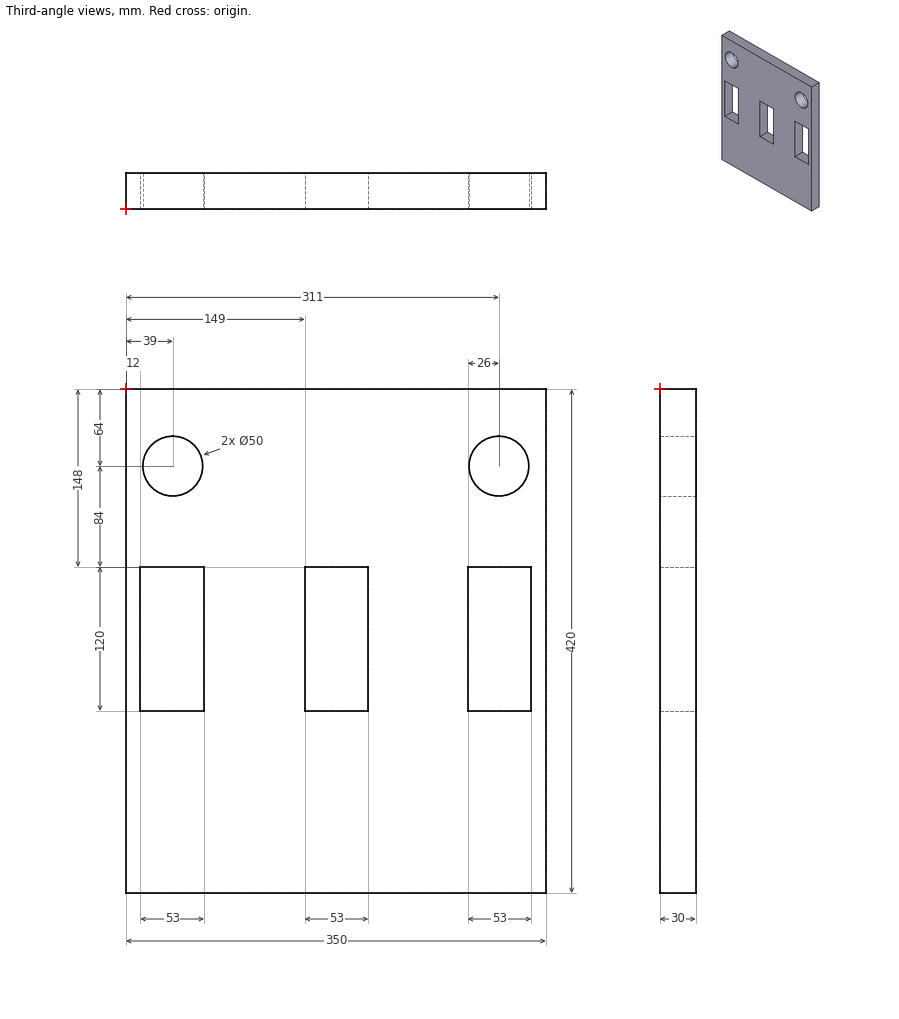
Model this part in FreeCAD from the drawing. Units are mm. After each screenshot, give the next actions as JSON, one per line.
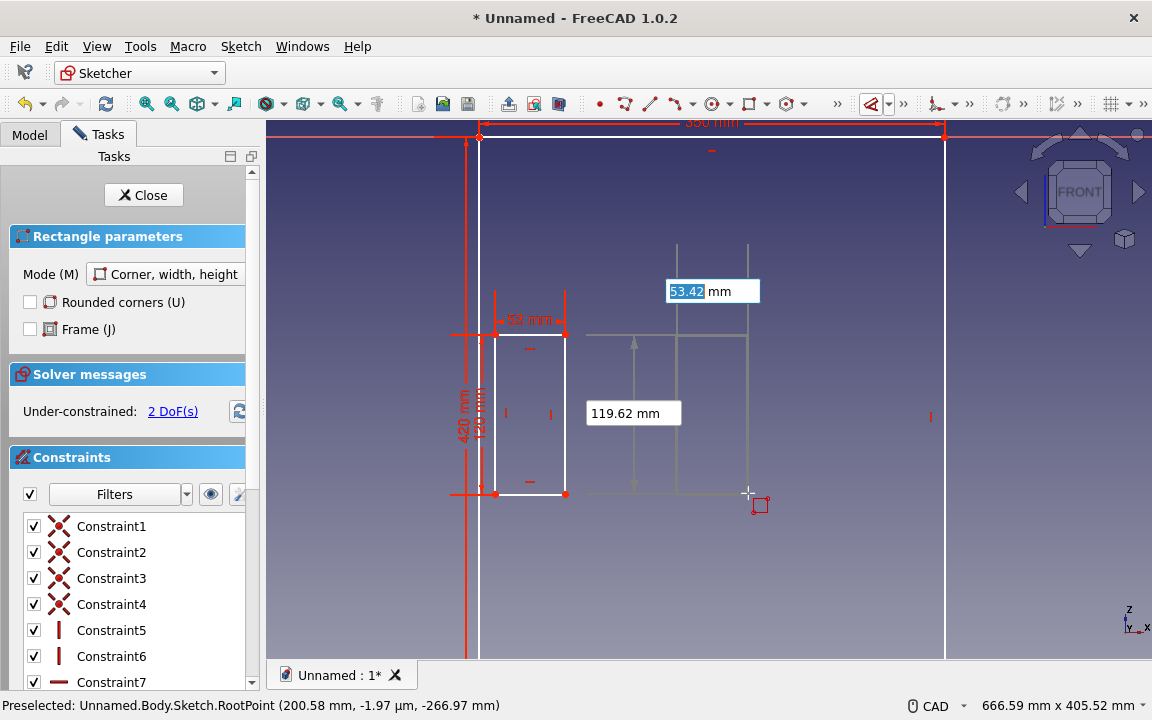
{"action": "type", "text": "53"}
{"action": "key", "text": "Tab"}
{"action": "type", "text": "120"}
{"action": "key", "text": "Return"}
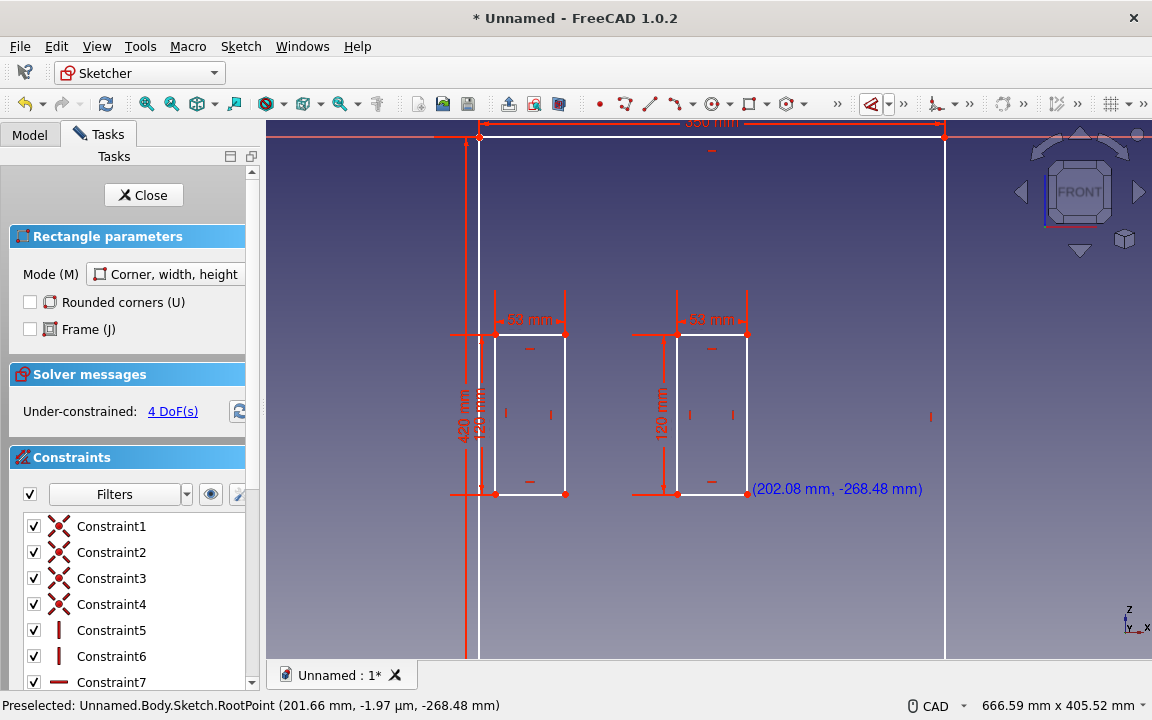
{"action": "left_click", "coordinate": [858, 334]}
{"action": "mouse_move", "coordinate": [929, 493]}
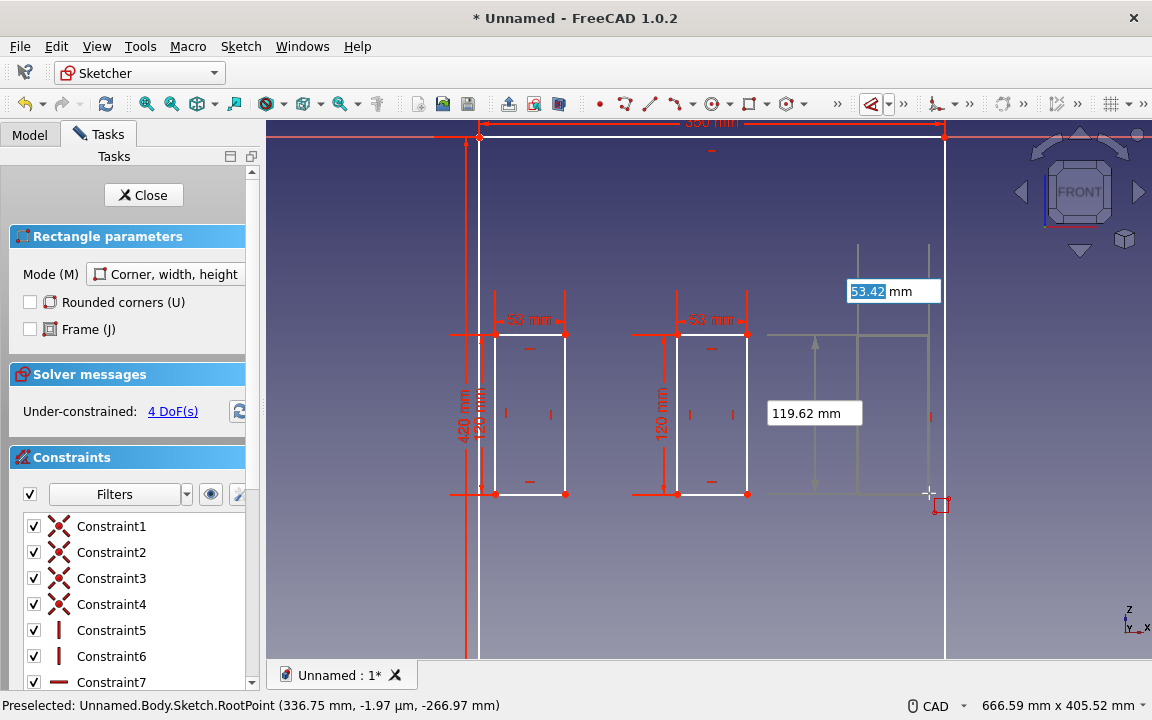
{"action": "type", "text": "53"}
{"action": "key", "text": "Tab"}
{"action": "type", "text": "120"}
{"action": "key", "text": "Return"}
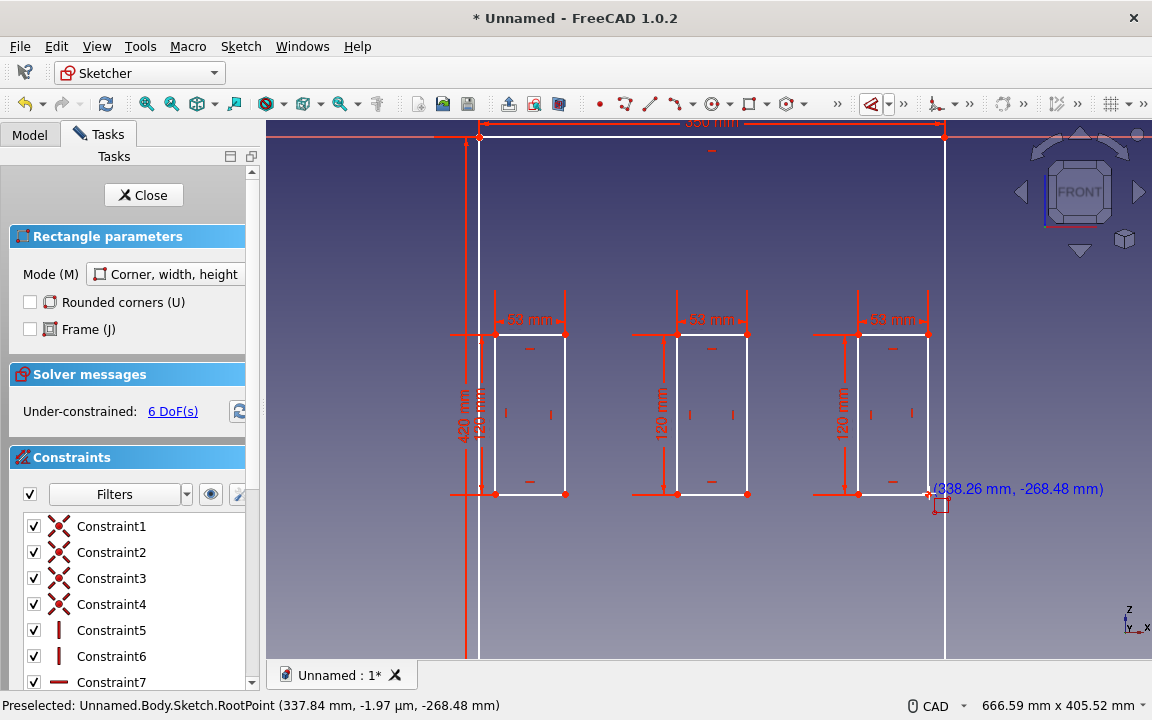
{"action": "left_click", "coordinate": [712, 104]}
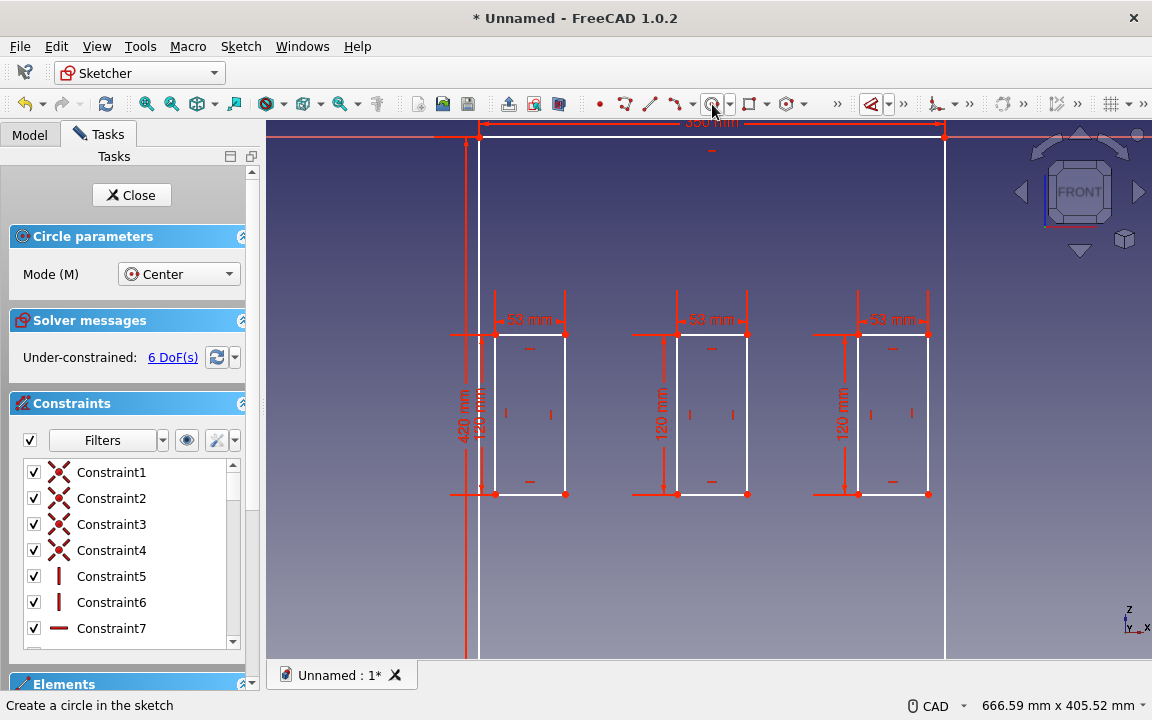
{"action": "left_click", "coordinate": [531, 222]}
{"action": "mouse_move", "coordinate": [555, 199]}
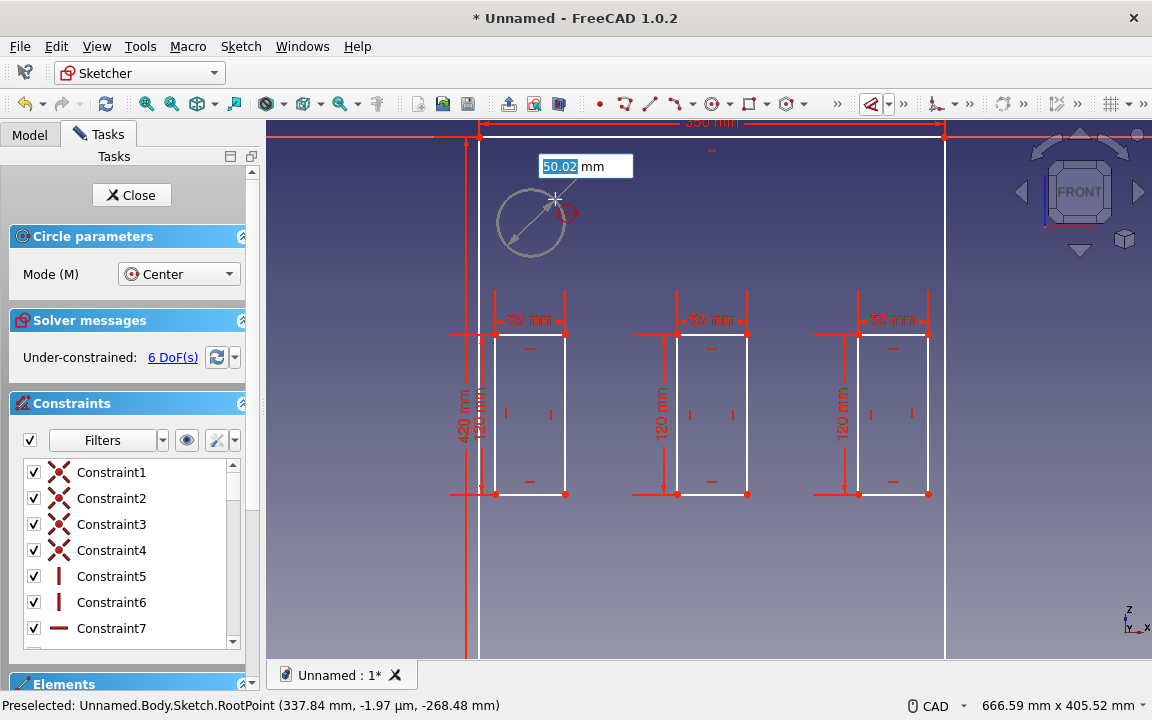
{"action": "type", "text": "50"}
{"action": "key", "text": "Return"}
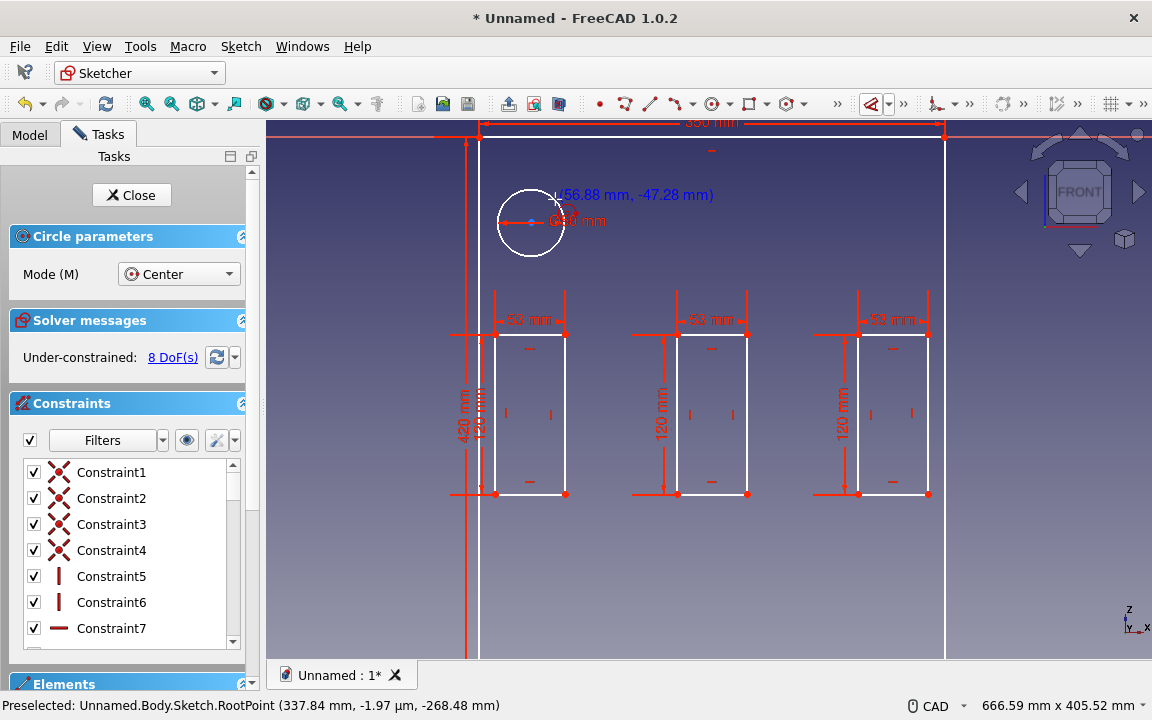
{"action": "left_click", "coordinate": [893, 222]}
{"action": "mouse_move", "coordinate": [916, 199]}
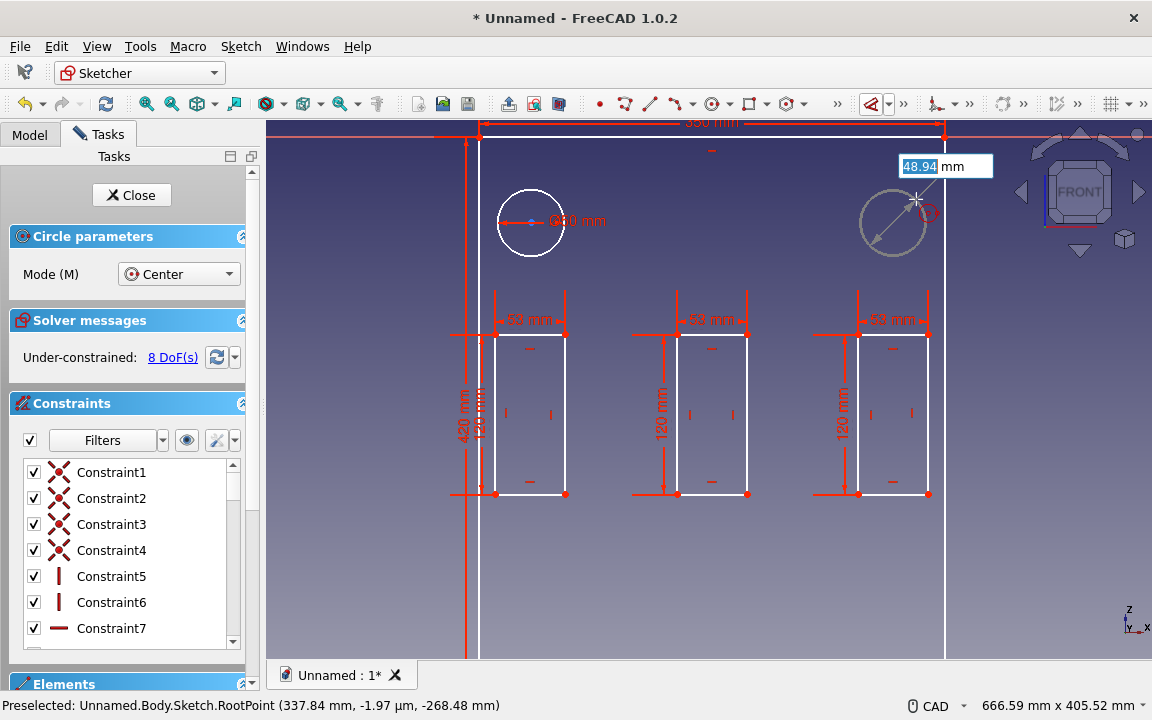
{"action": "type", "text": "50"}
{"action": "key", "text": "Return"}
{"action": "key", "text": "Escape"}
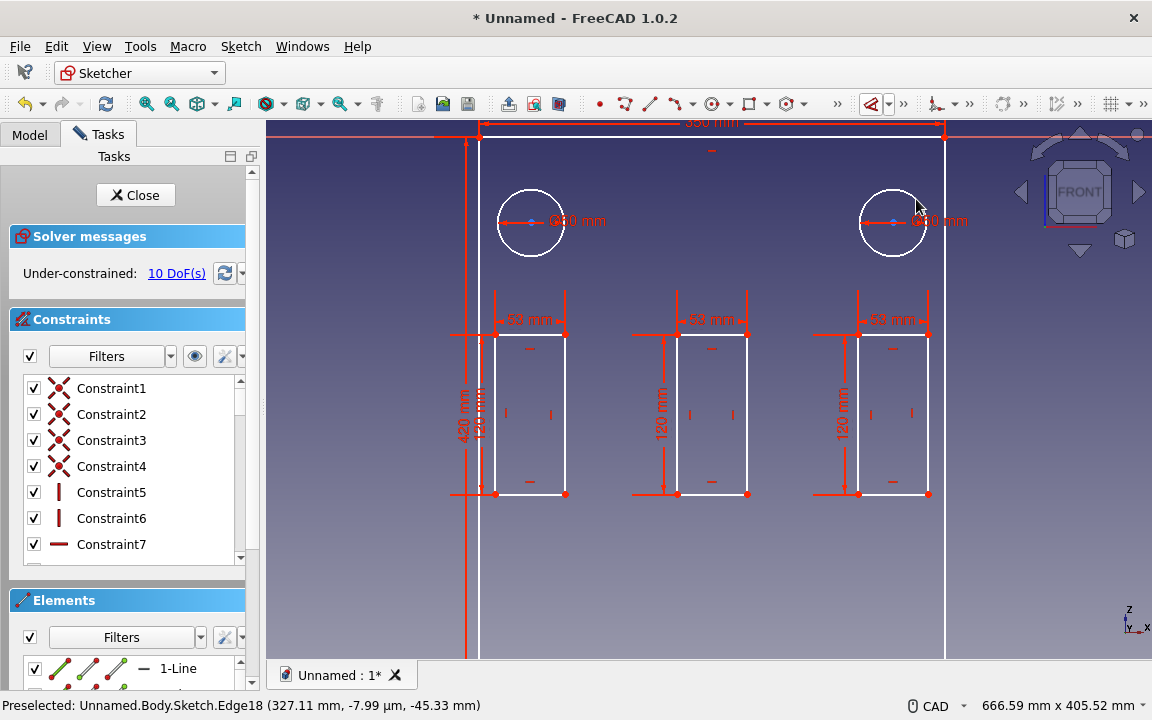
{"action": "left_click", "coordinate": [870, 104]}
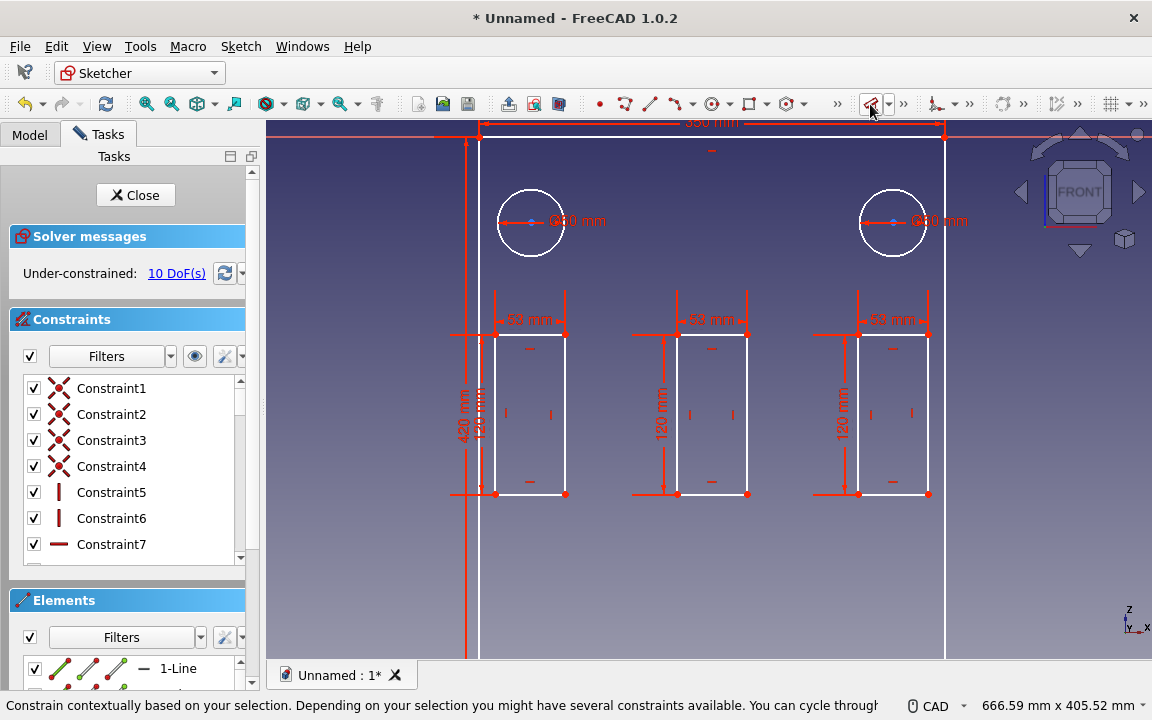
{"action": "left_click", "coordinate": [531, 223]}
{"action": "left_click", "coordinate": [493, 257]}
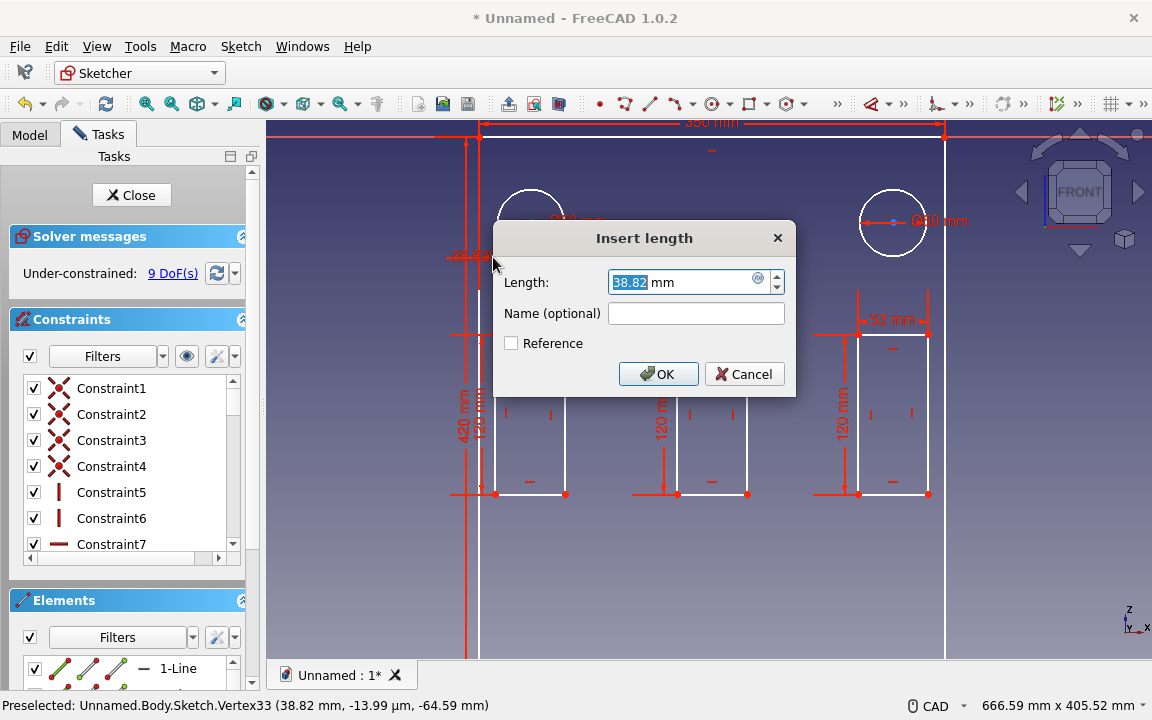
{"action": "type", "text": "39"}
{"action": "key", "text": "Return"}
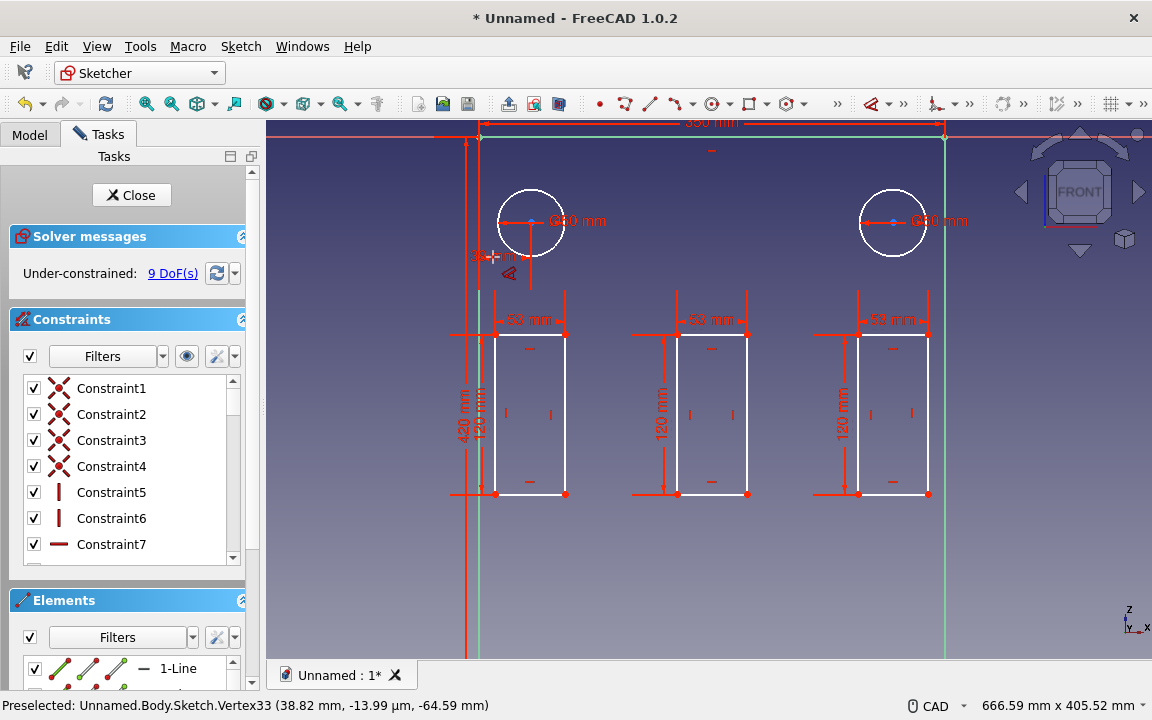
{"action": "left_click", "coordinate": [531, 223]}
{"action": "left_click", "coordinate": [445, 186]}